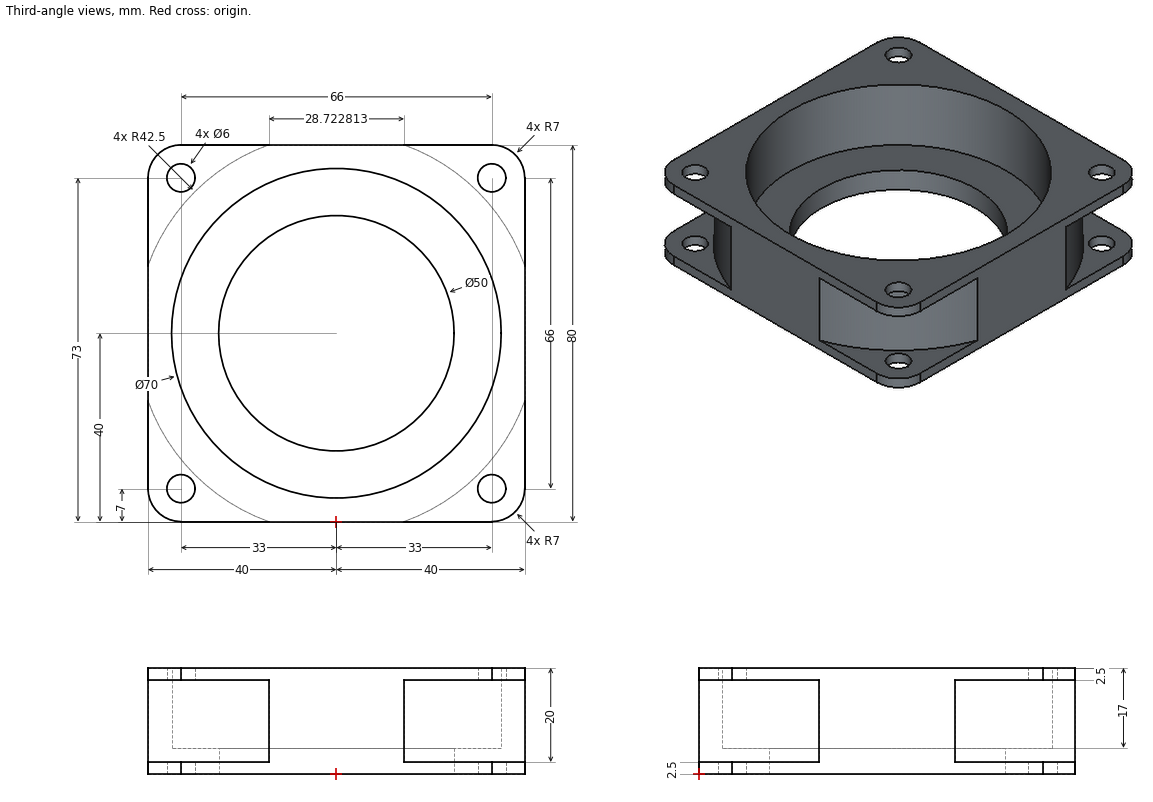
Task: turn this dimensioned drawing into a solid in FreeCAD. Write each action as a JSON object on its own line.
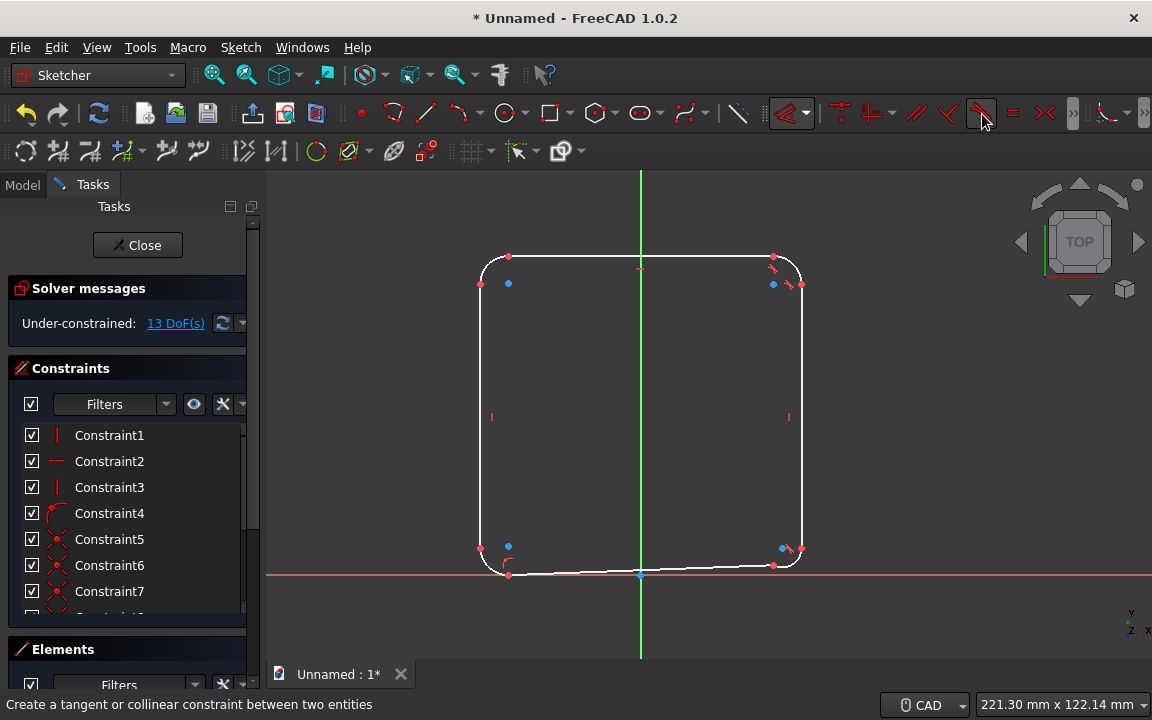
{"action": "left_click", "coordinate": [694, 256]}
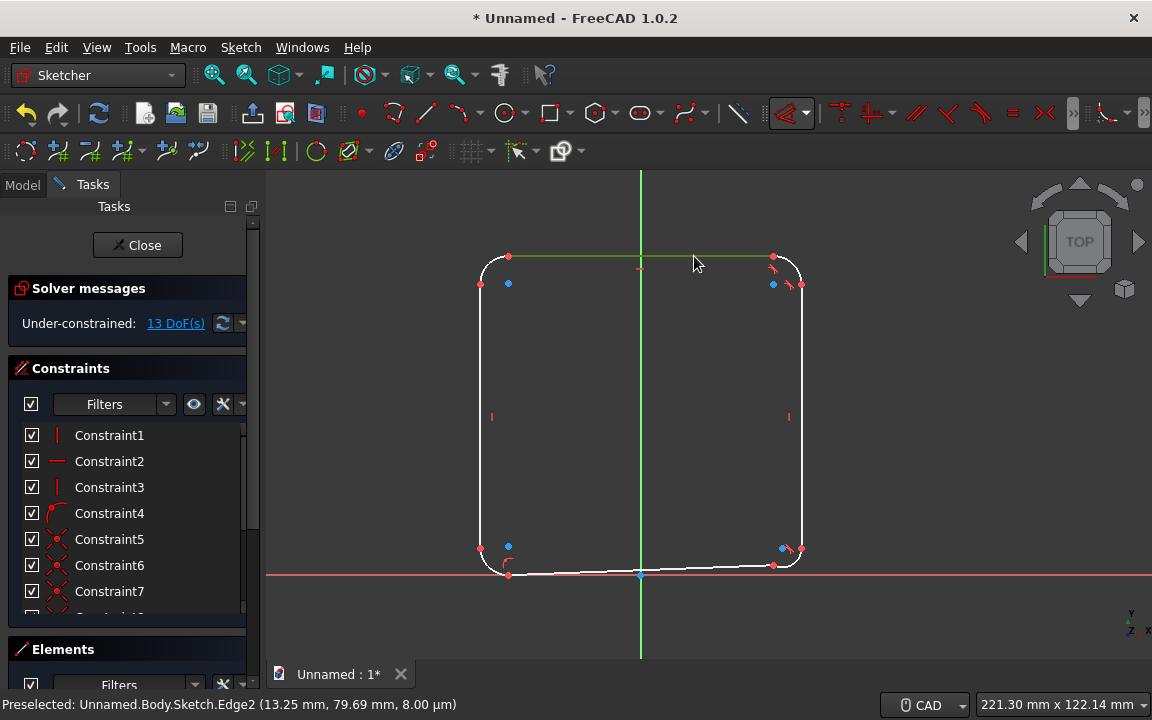
{"action": "left_click", "coordinate": [496, 259]}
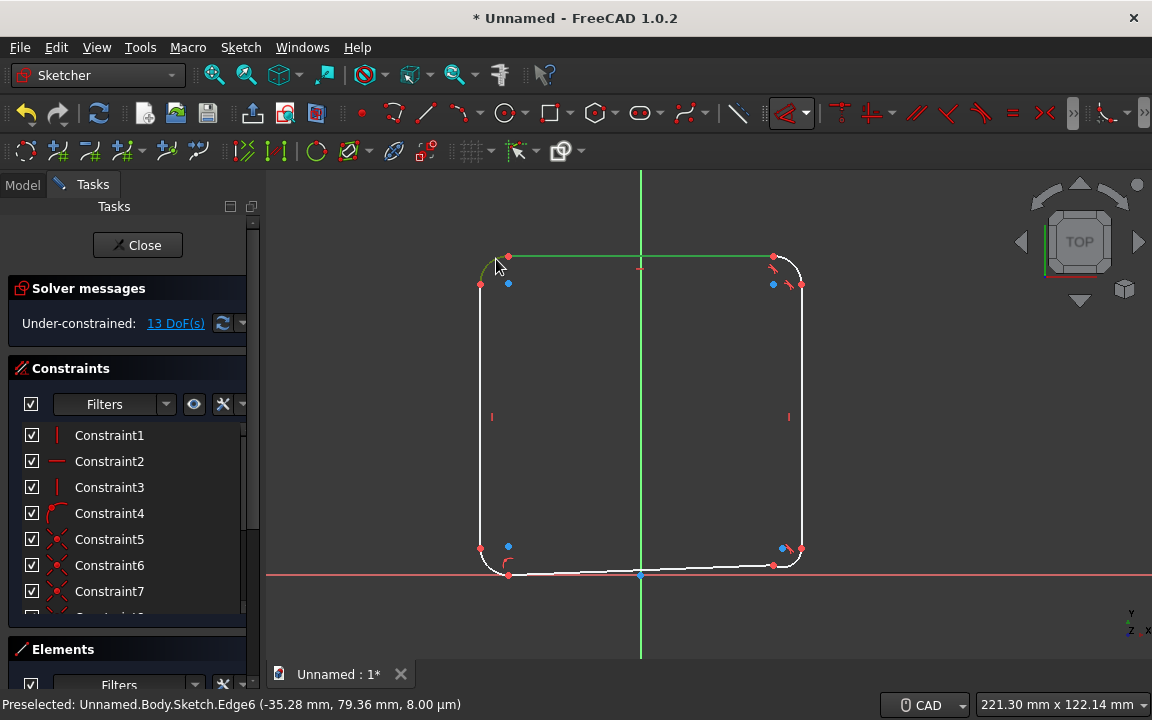
{"action": "left_click", "coordinate": [982, 114]}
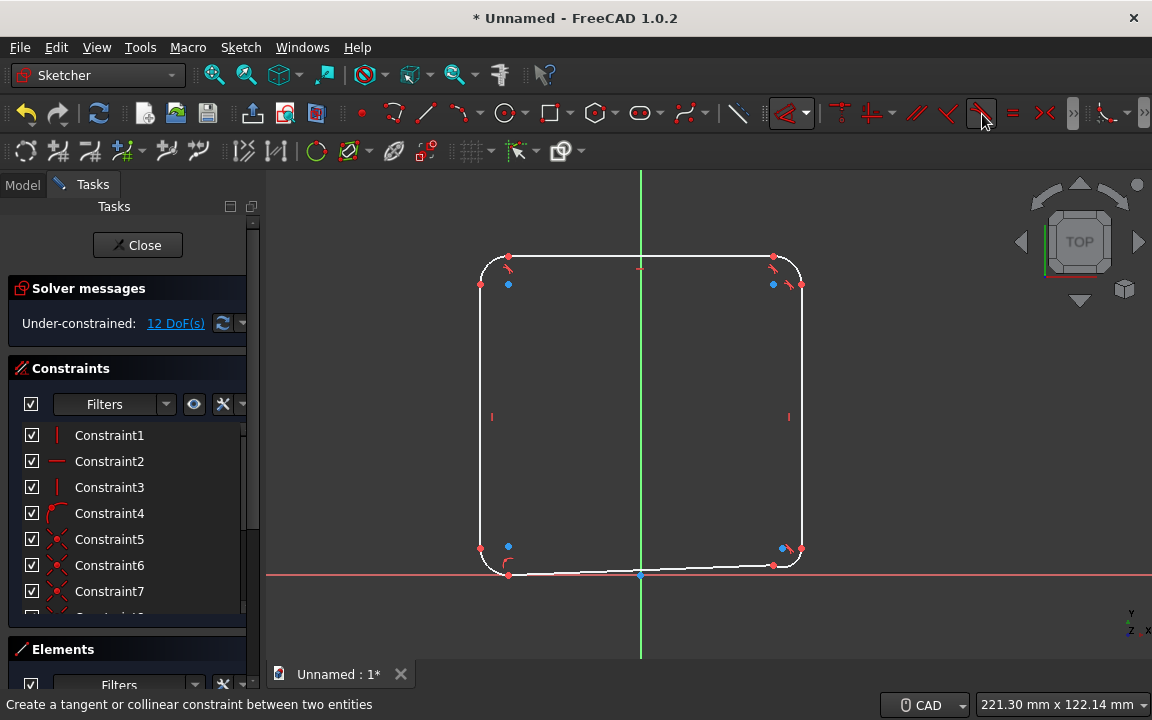
{"action": "left_click", "coordinate": [480, 363]}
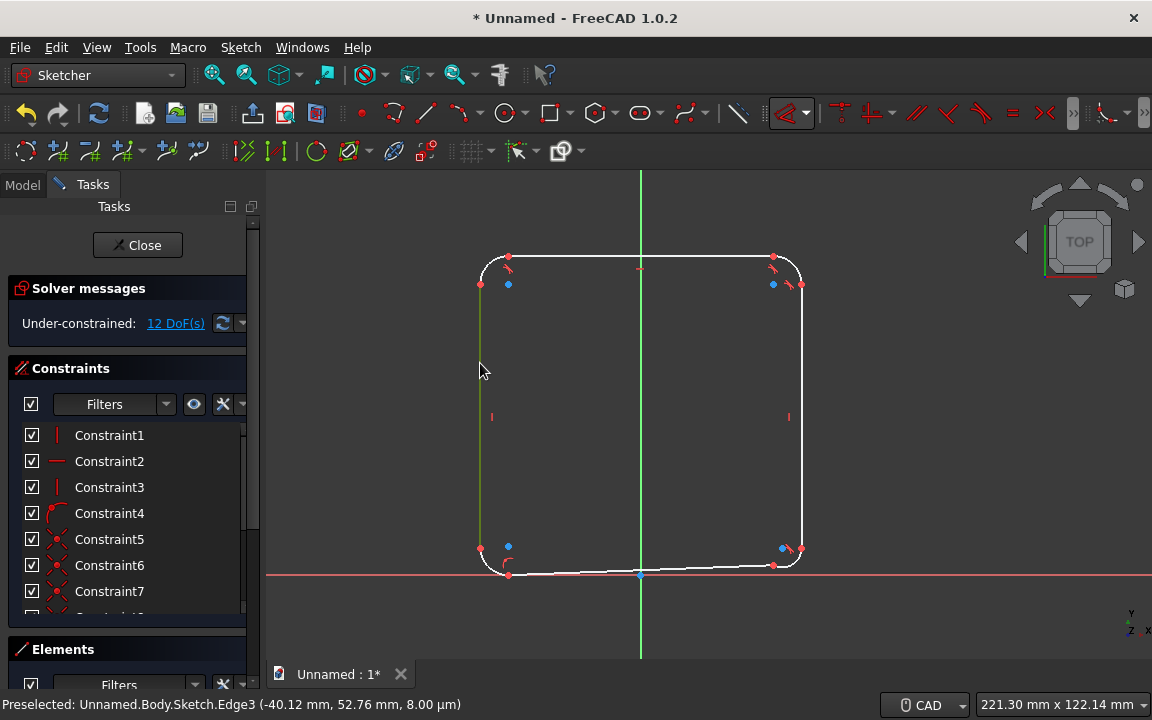
{"action": "left_click", "coordinate": [496, 259]}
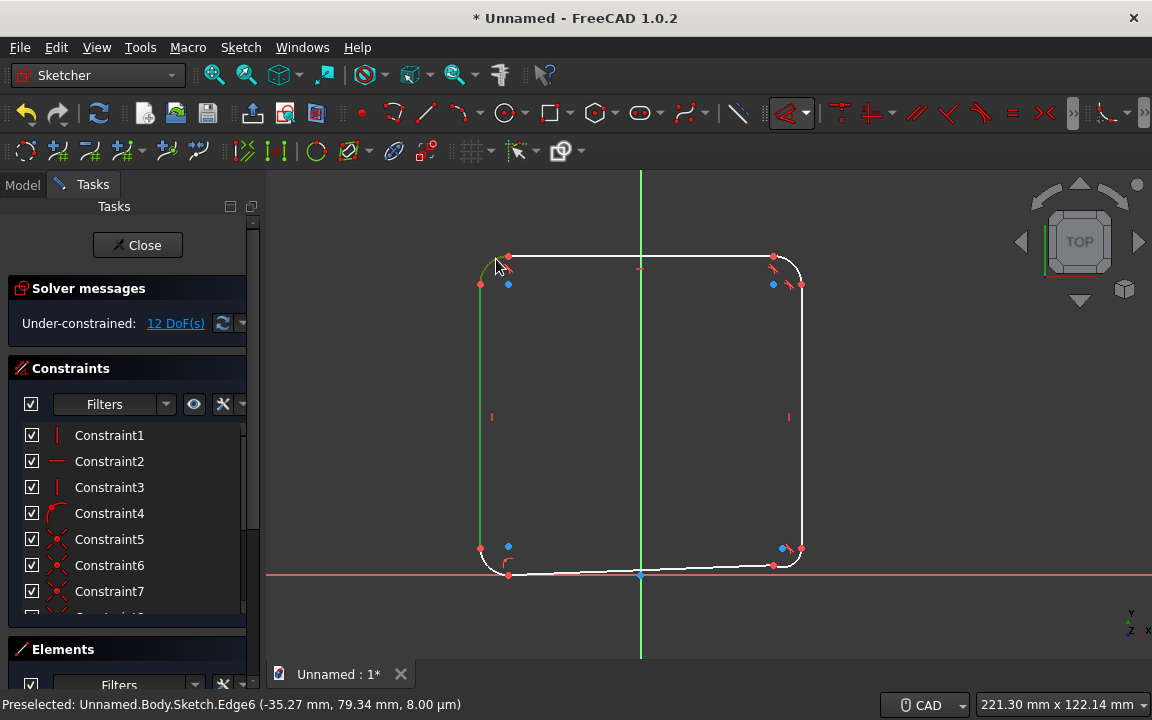
{"action": "key", "text": "t"}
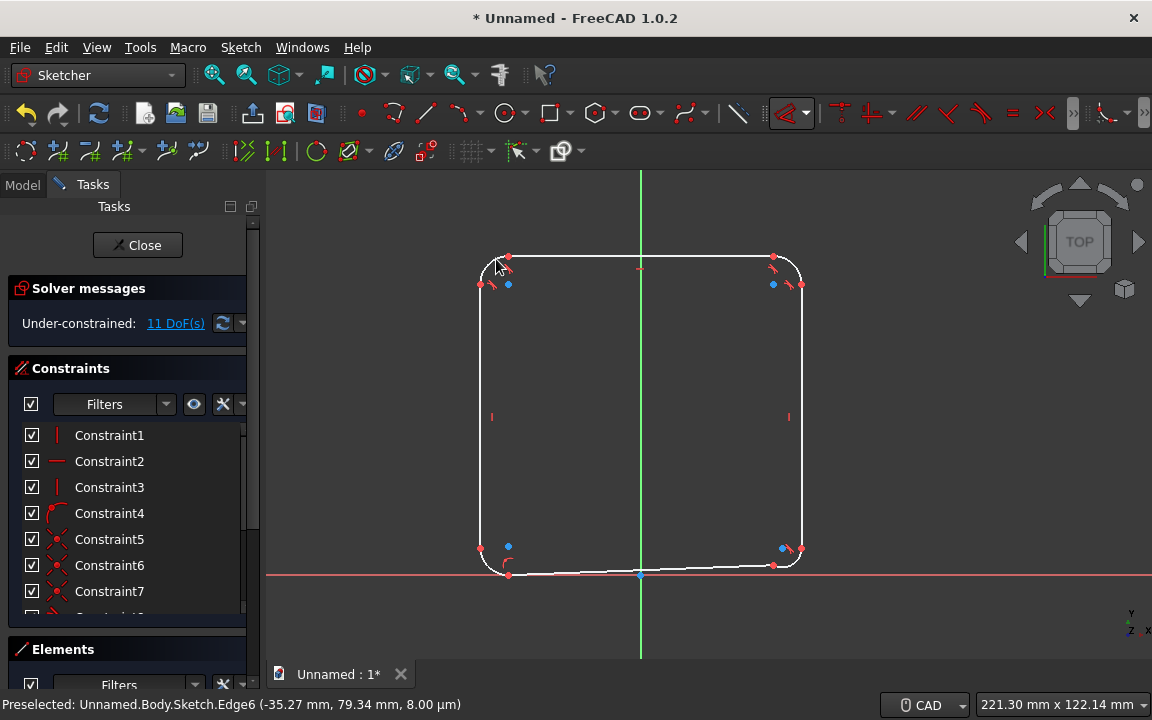
{"action": "left_click", "coordinate": [480, 363]}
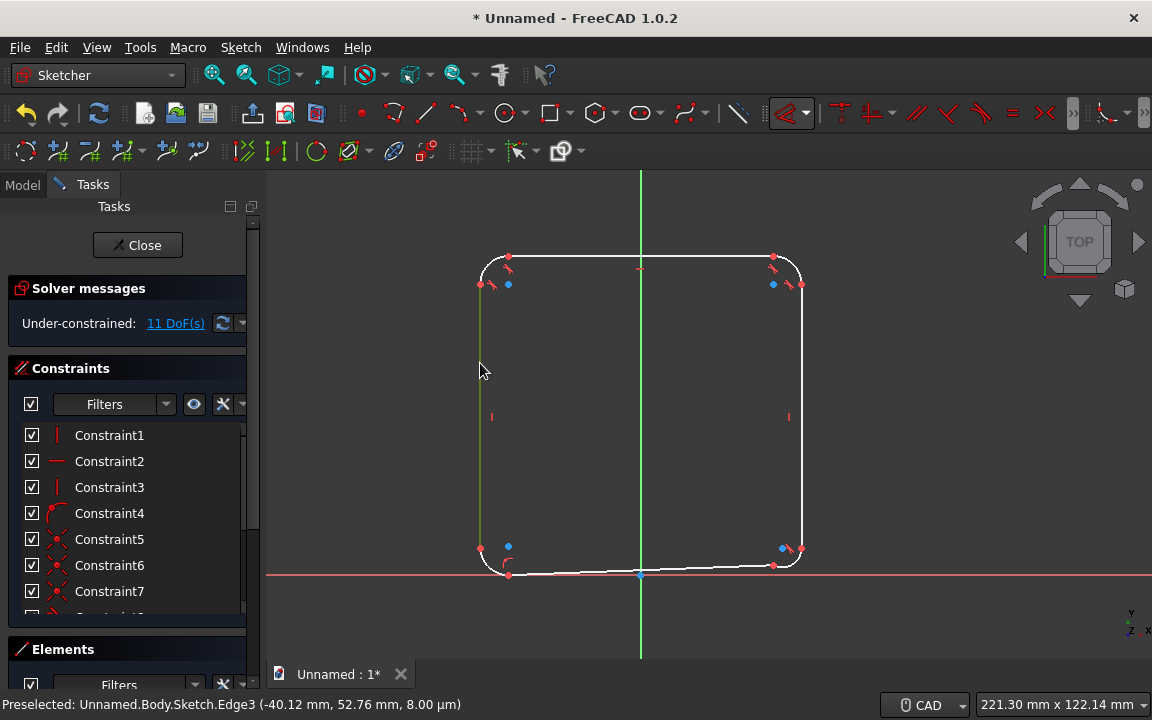
{"action": "left_click", "coordinate": [484, 560]}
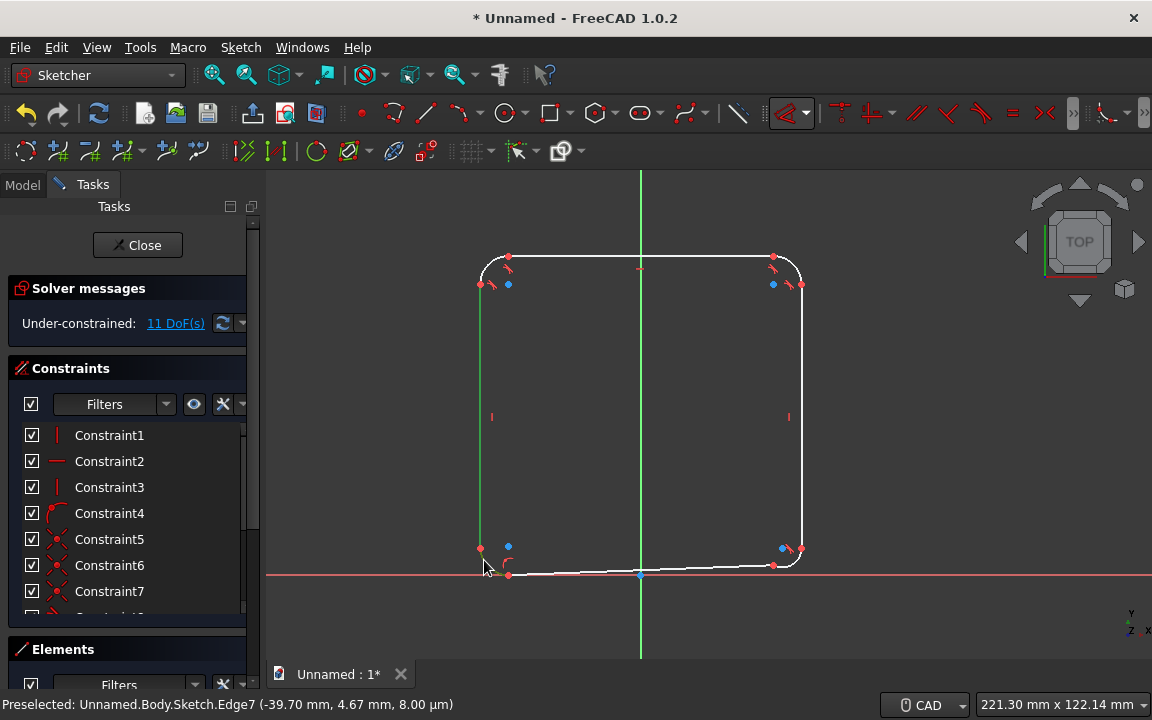
{"action": "left_click", "coordinate": [982, 114]}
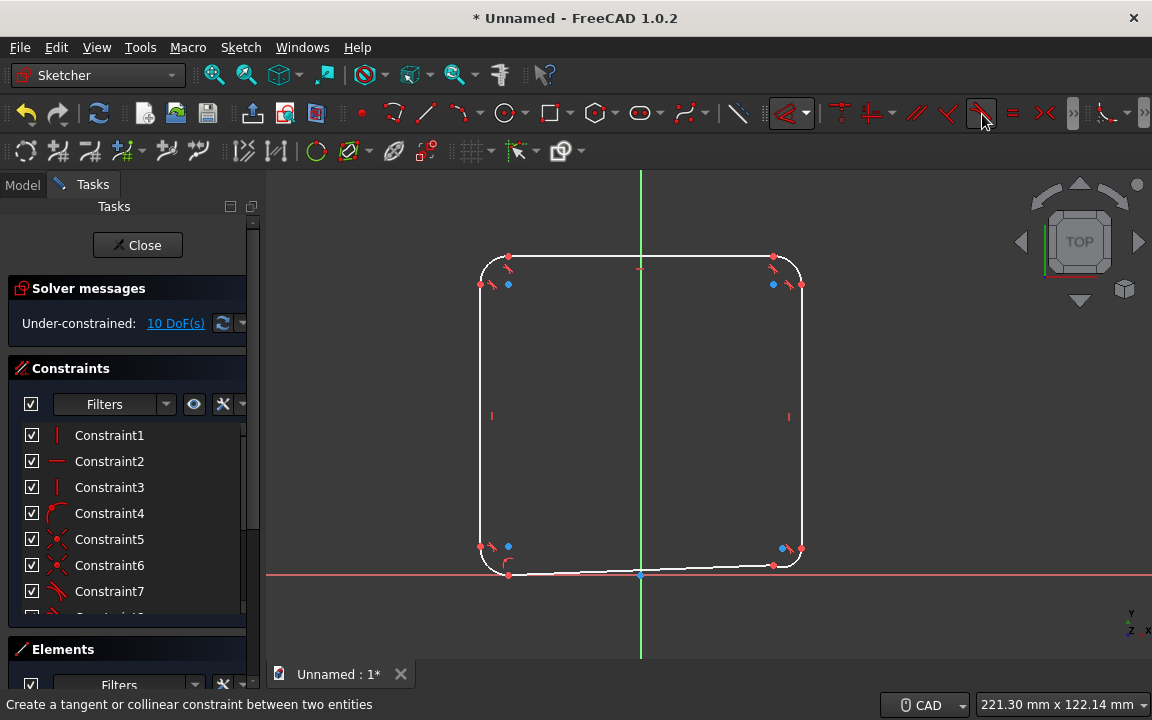
{"action": "left_click", "coordinate": [588, 572]}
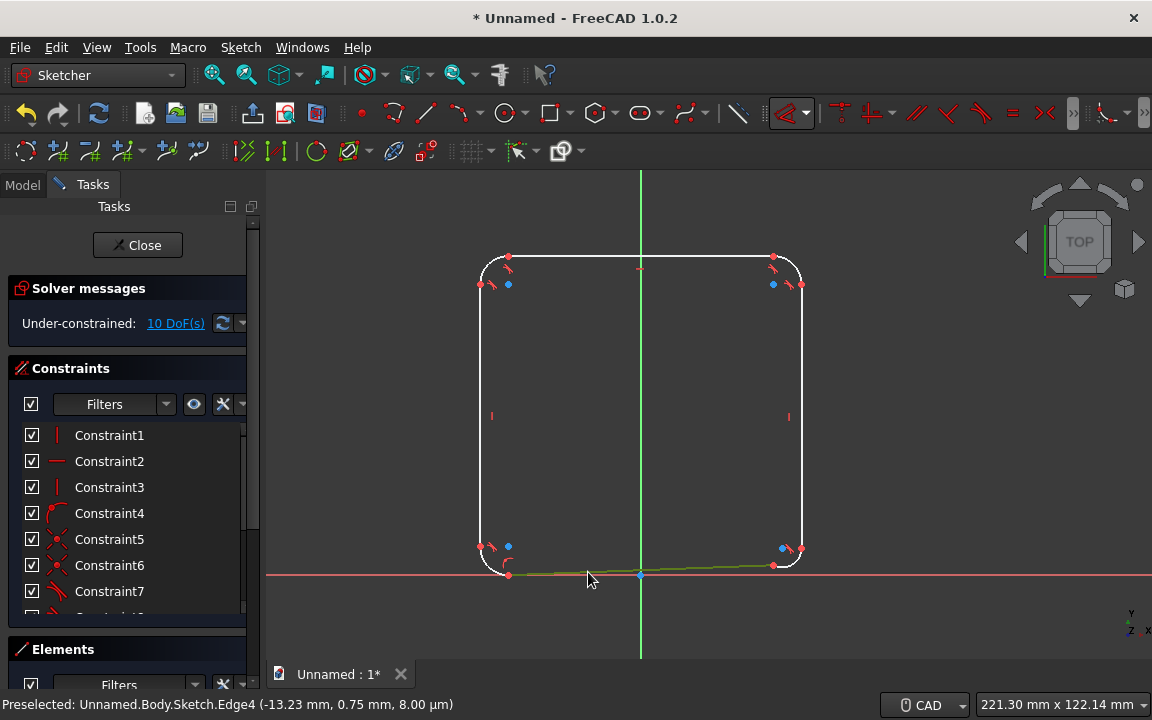
{"action": "left_click", "coordinate": [483, 560]}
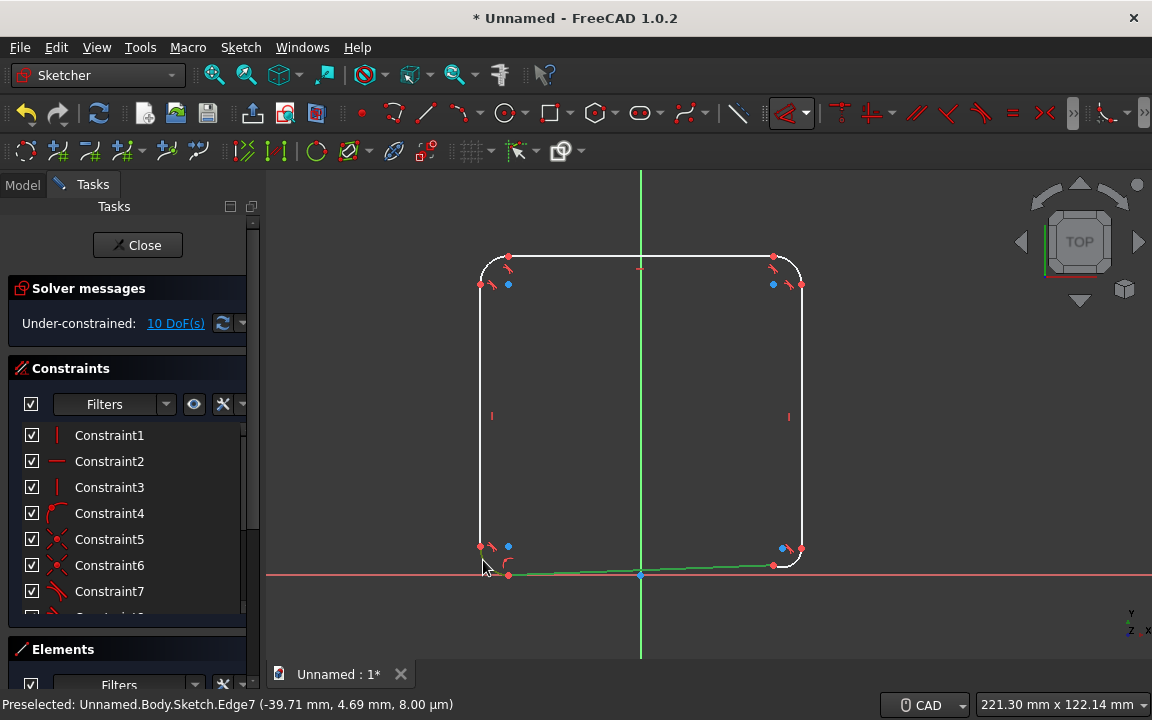
{"action": "key", "text": "t"}